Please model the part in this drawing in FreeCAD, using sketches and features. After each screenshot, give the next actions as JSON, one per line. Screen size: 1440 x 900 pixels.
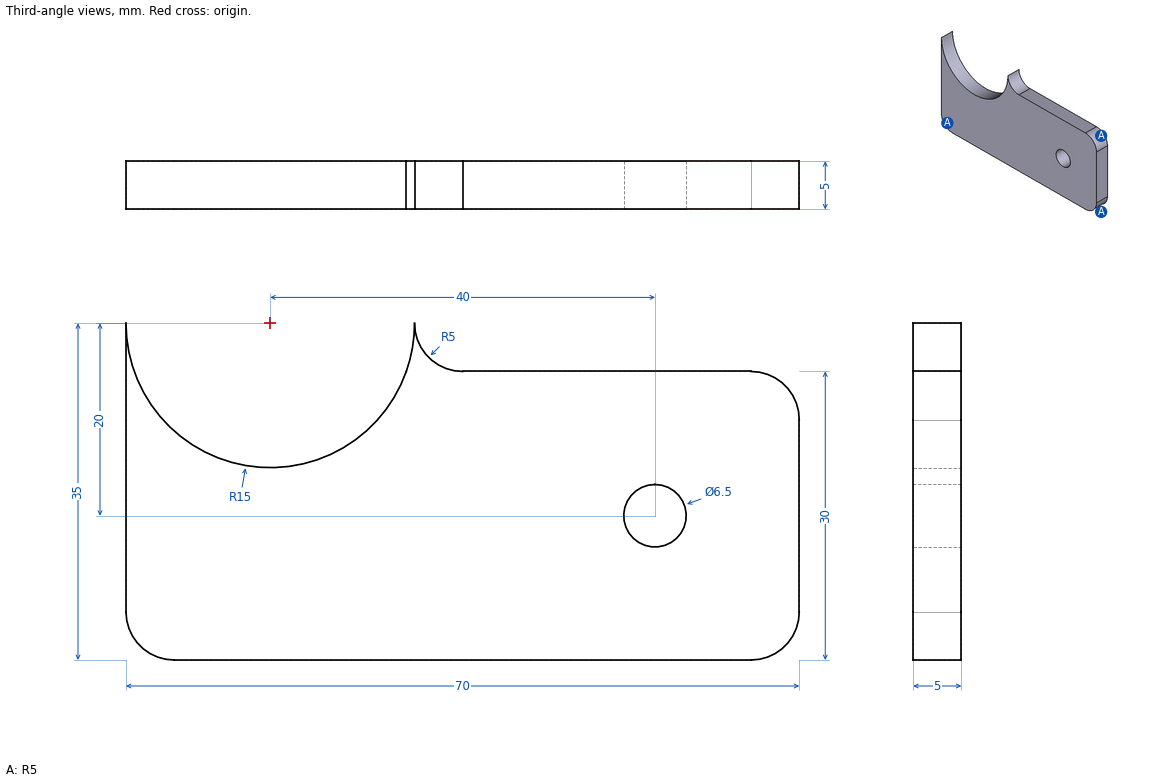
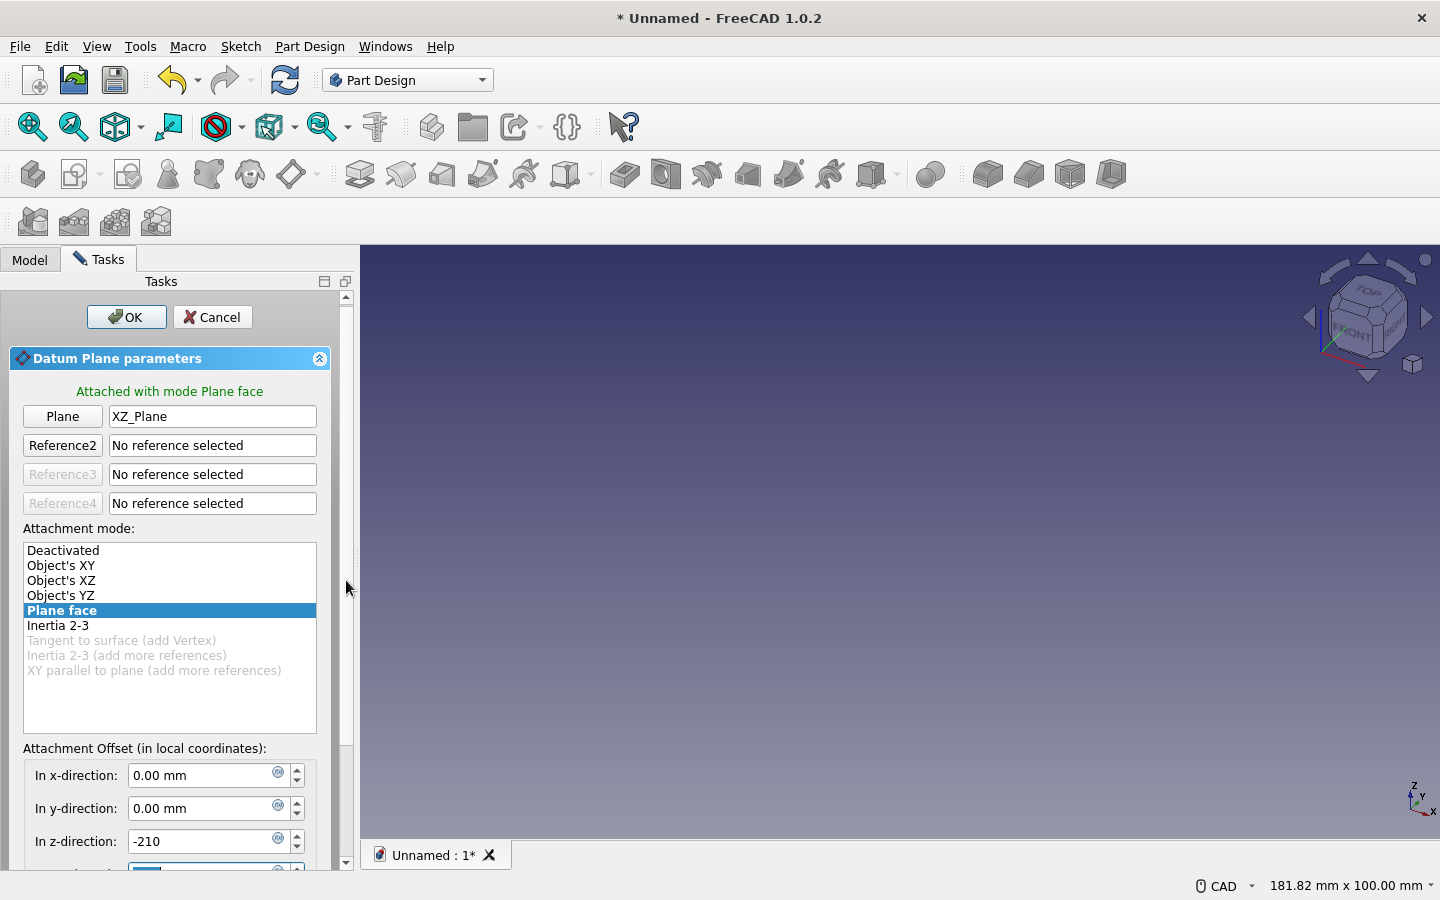
{"action": "left_click", "coordinate": [127, 320]}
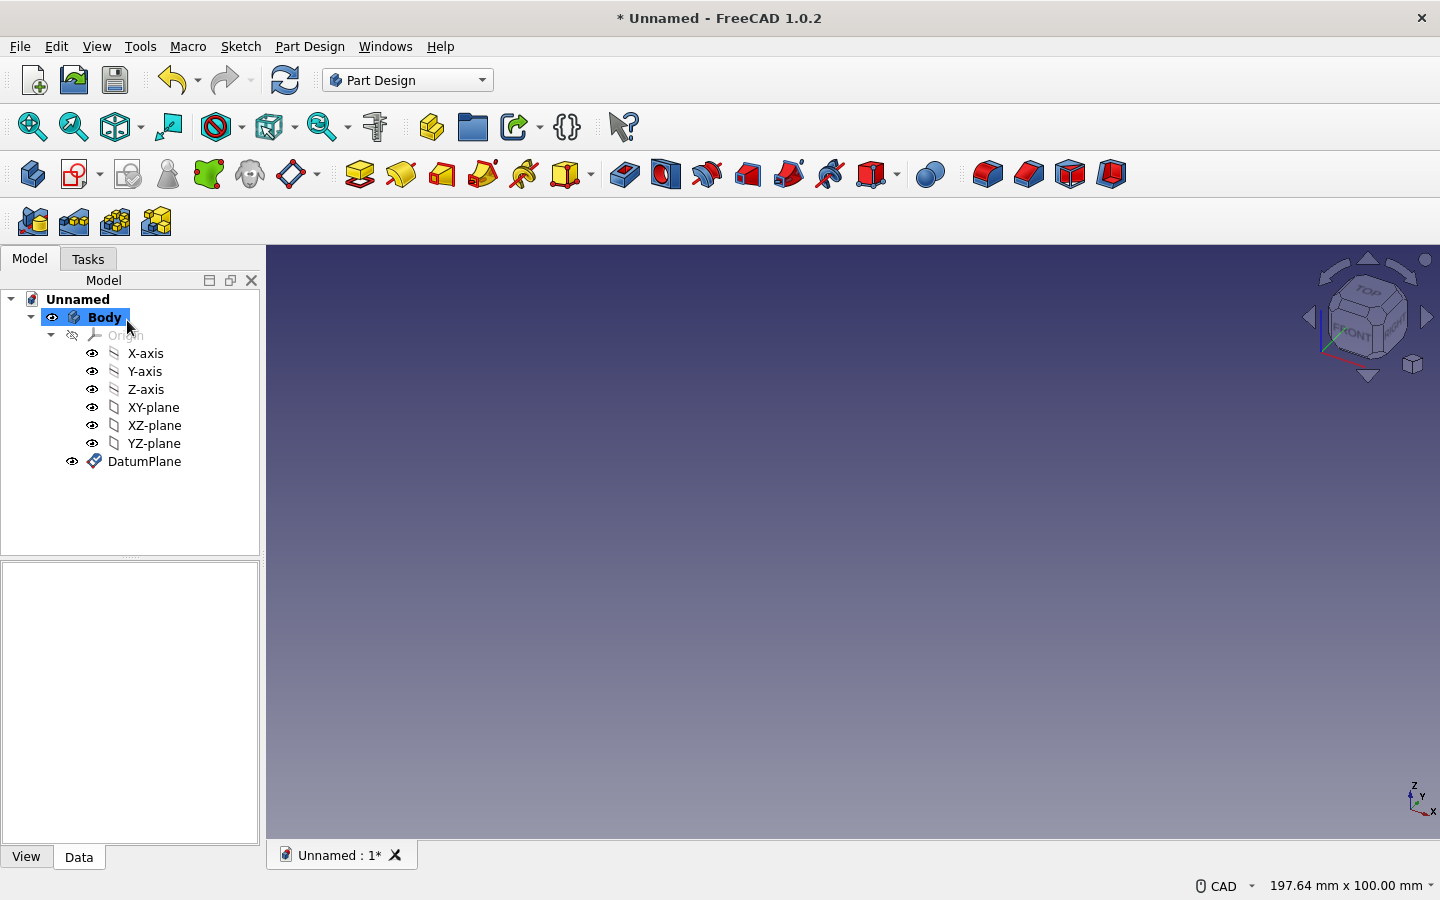
{"action": "left_click", "coordinate": [117, 461]}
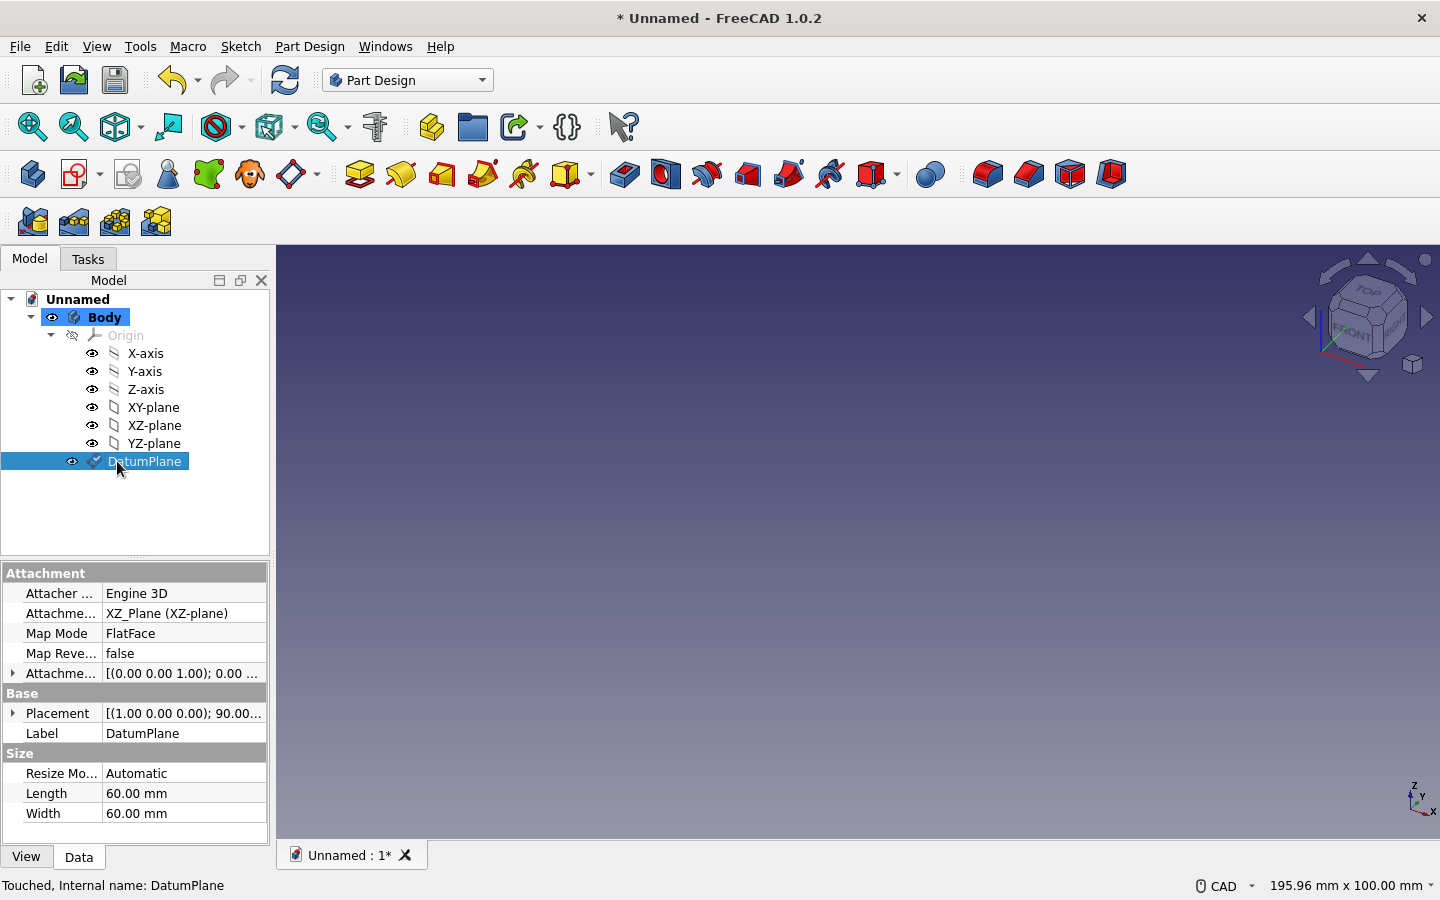
{"action": "left_click", "coordinate": [74, 174]}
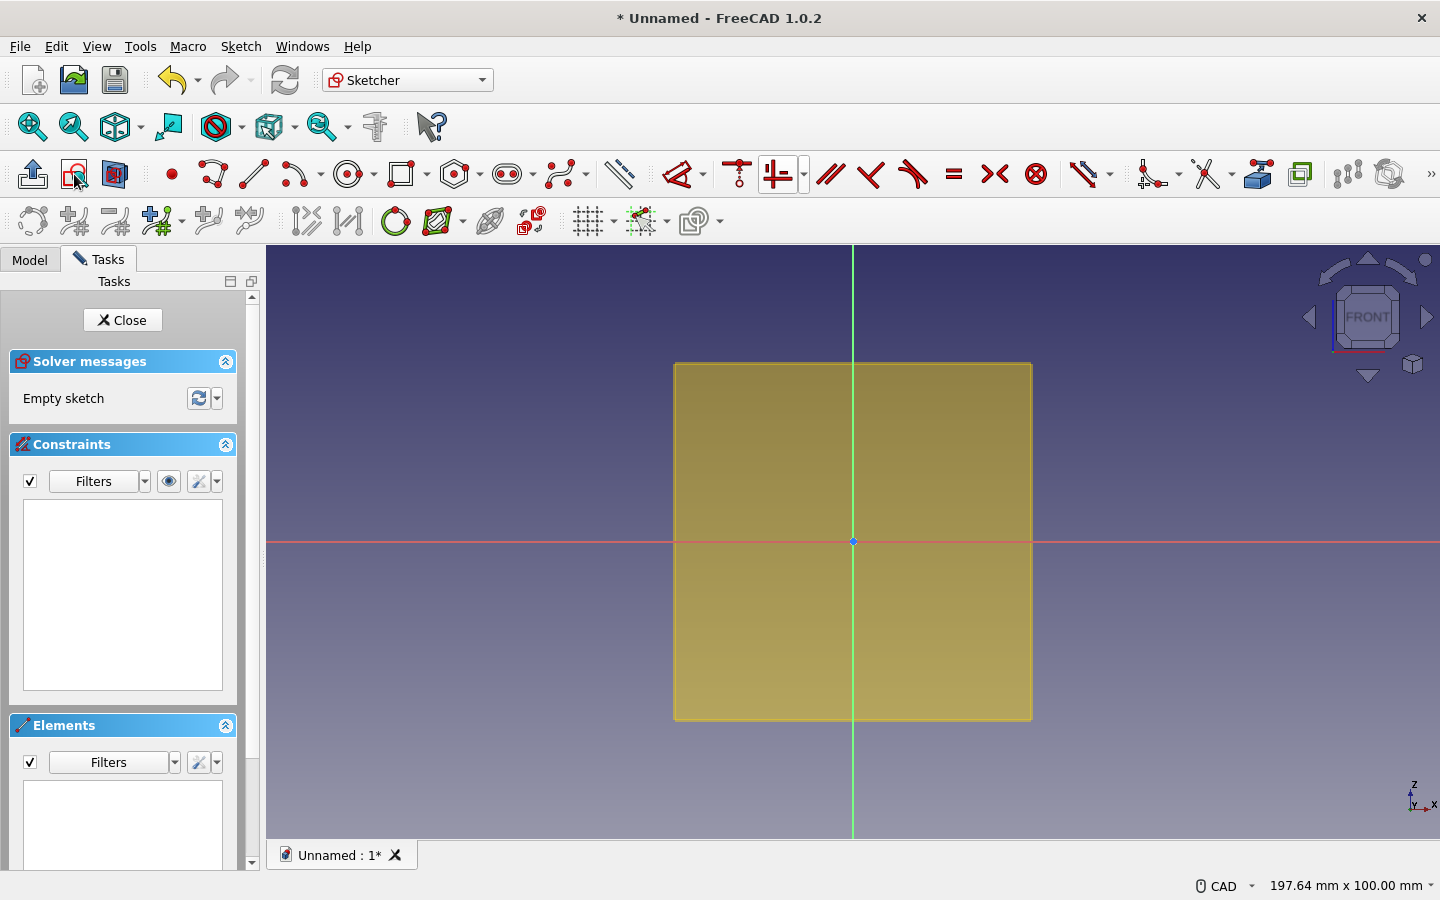
{"action": "scroll", "coordinate": [1200, 772], "scroll_direction": "up", "scroll_amount": 3}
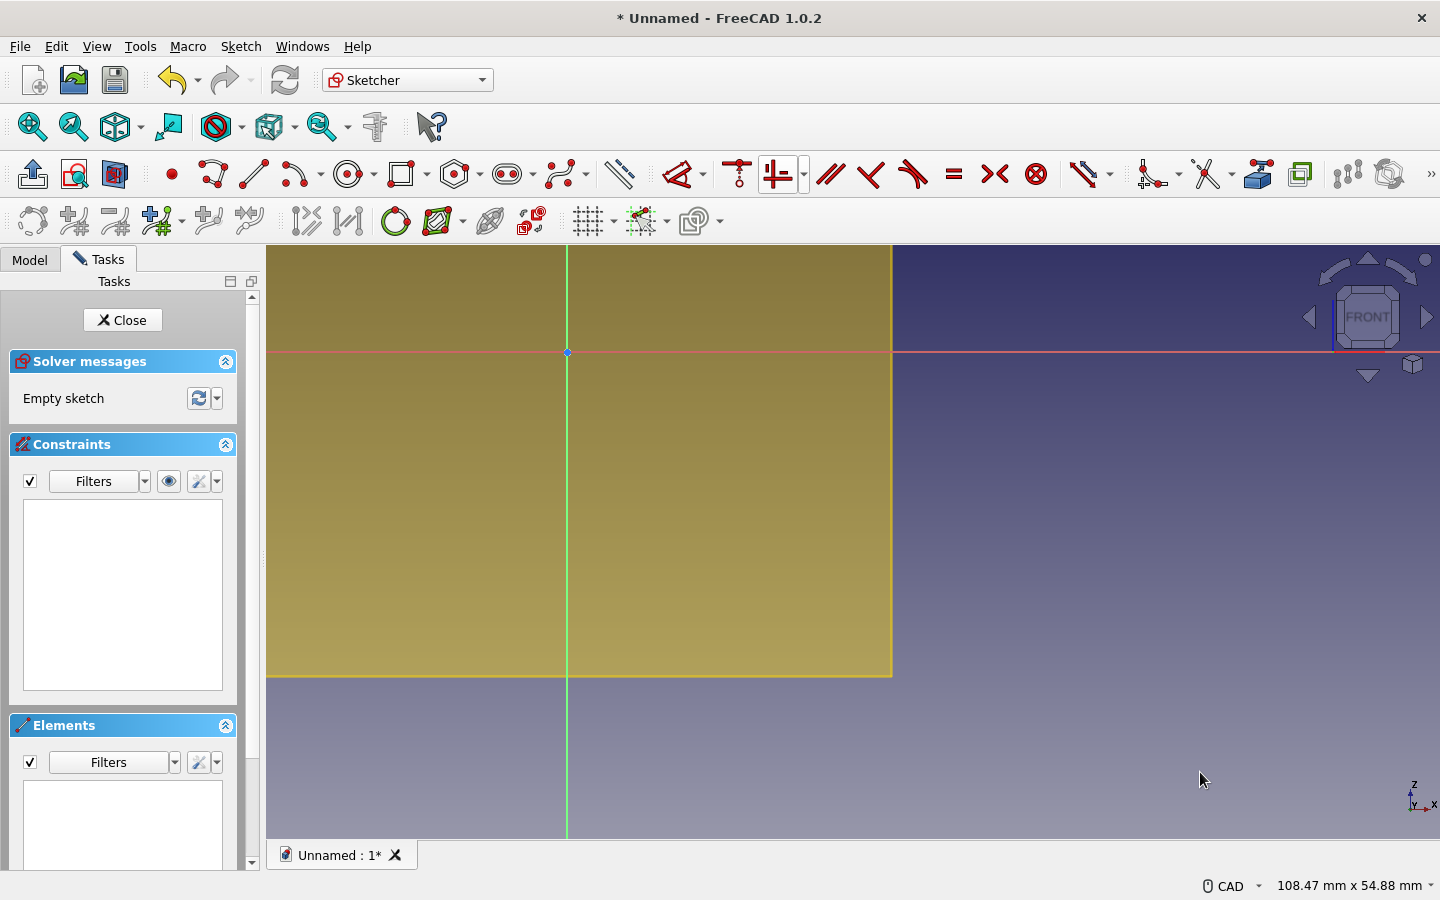
{"action": "left_click", "coordinate": [213, 174]}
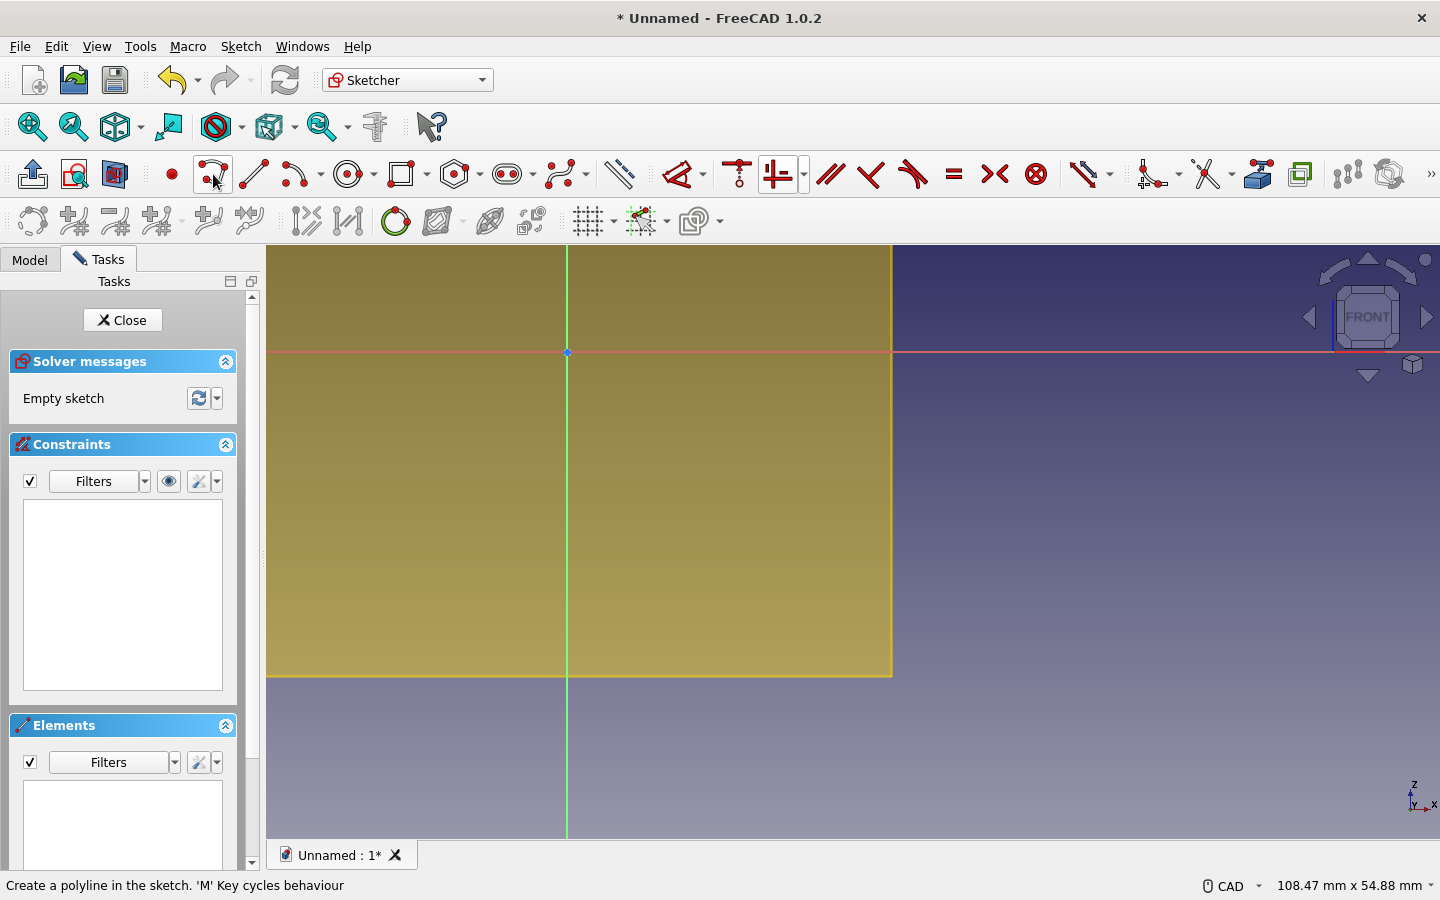
{"action": "left_click", "coordinate": [720, 406]}
{"action": "left_click", "coordinate": [1162, 406]}
{"action": "left_click", "coordinate": [1162, 731]}
{"action": "left_click", "coordinate": [405, 731]}
{"action": "left_click", "coordinate": [405, 352]}
{"action": "right_click", "coordinate": [405, 352]}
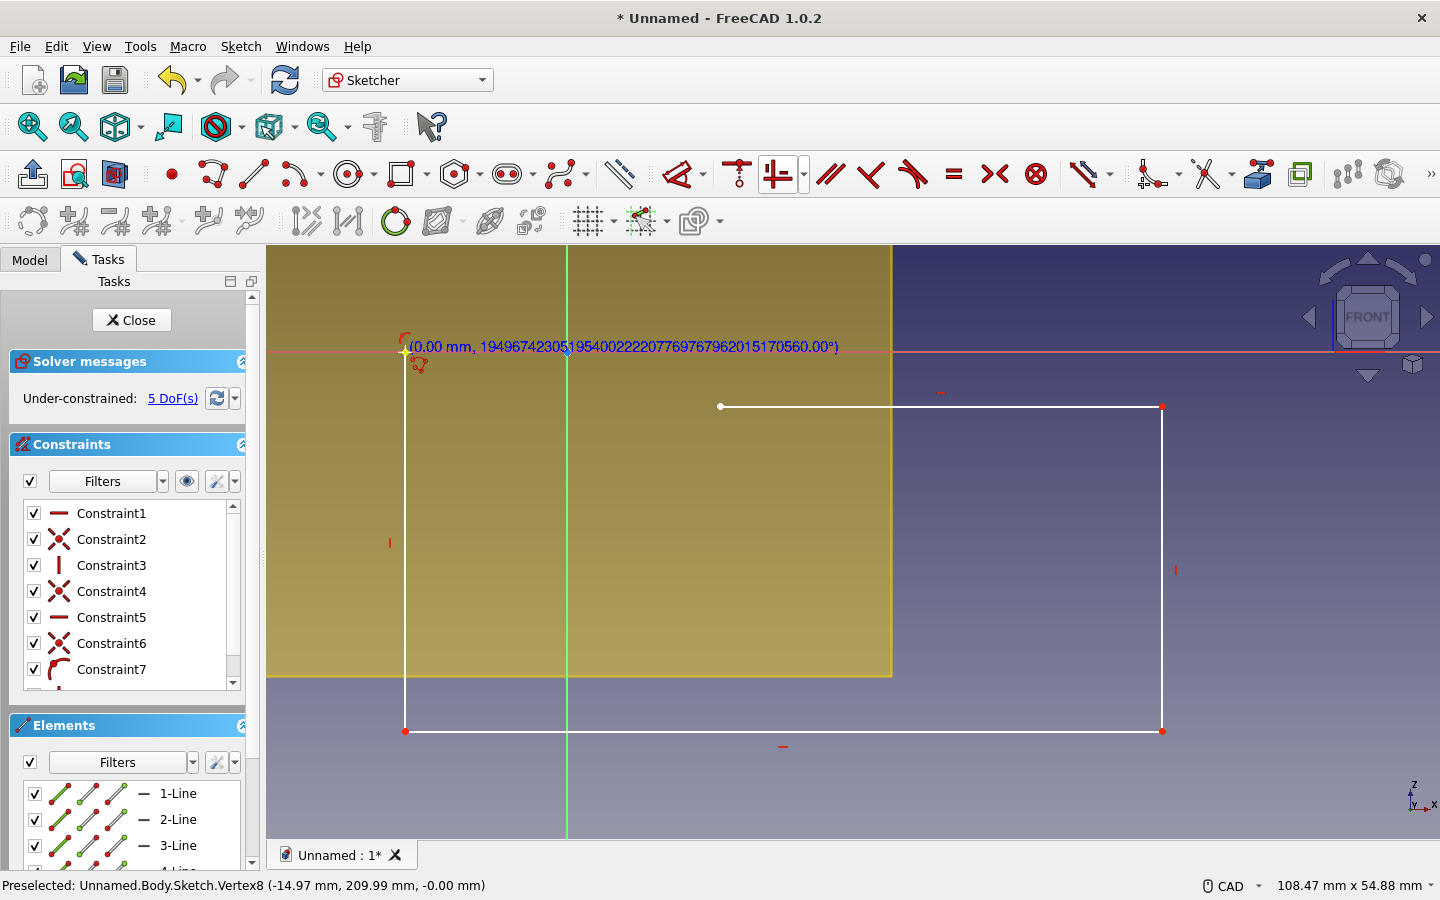
{"action": "key", "text": "g 3 a"}